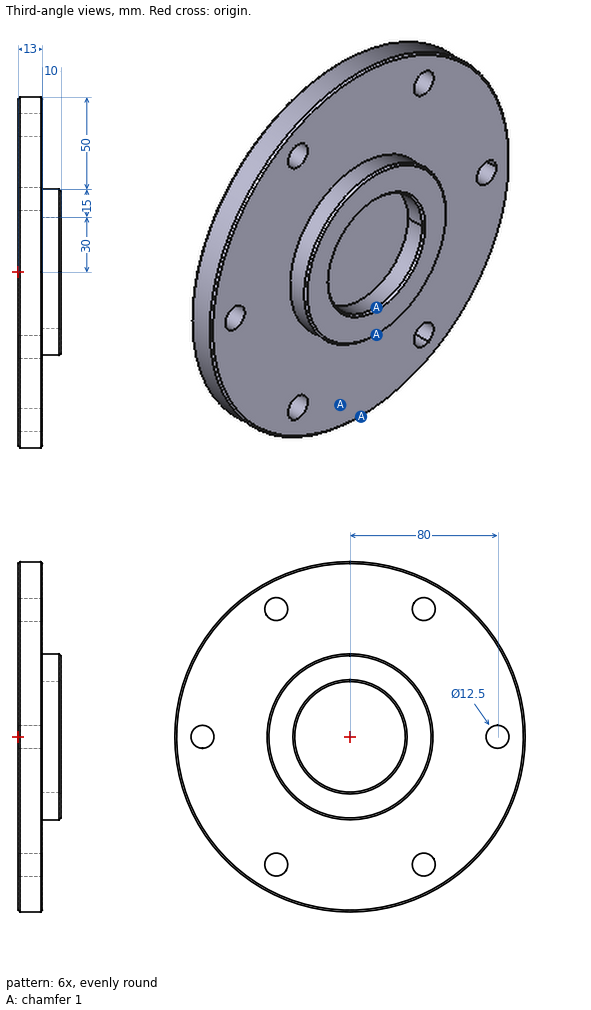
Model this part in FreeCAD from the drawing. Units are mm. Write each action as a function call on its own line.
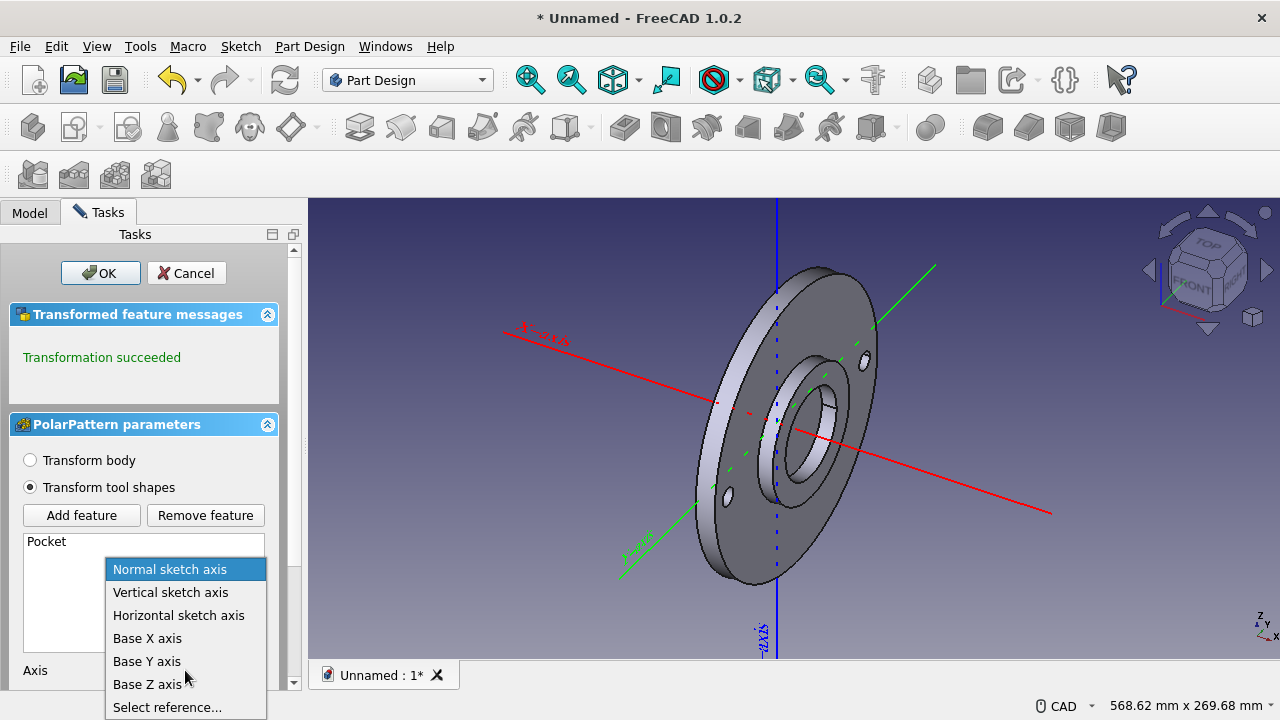
click(184, 638)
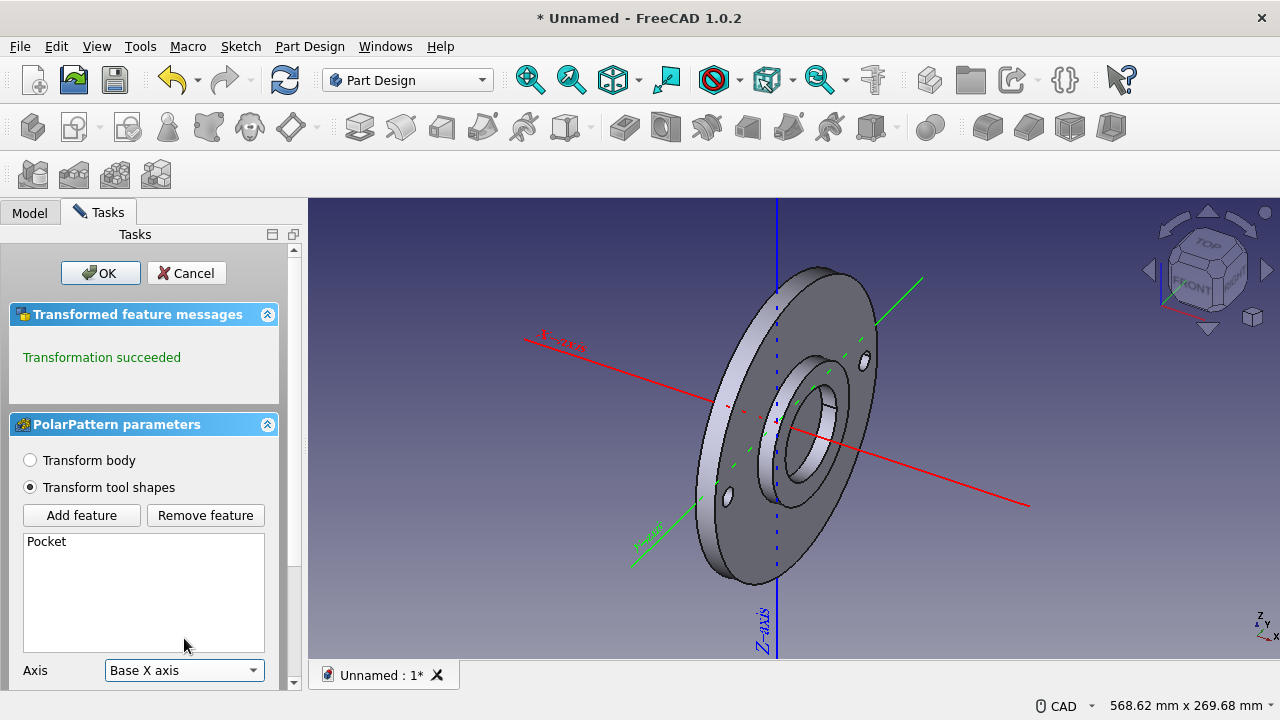
scroll(294, 467, down, 3)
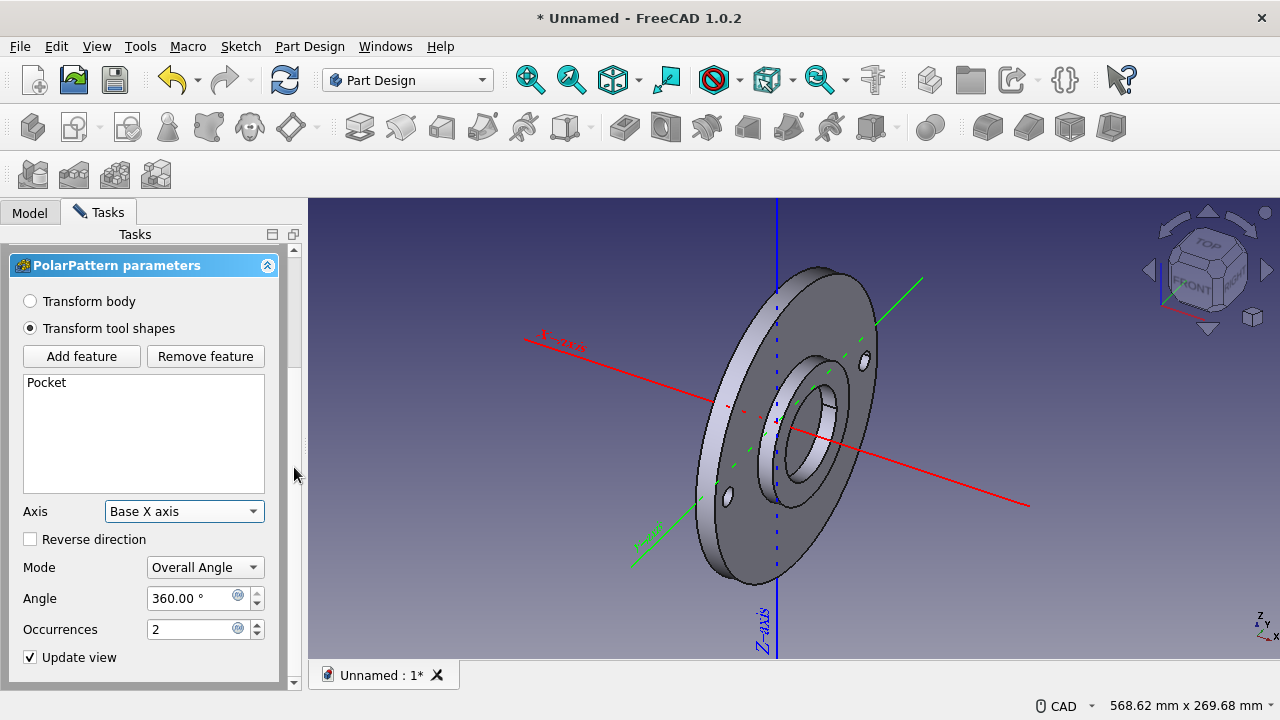
triple_click(199, 630)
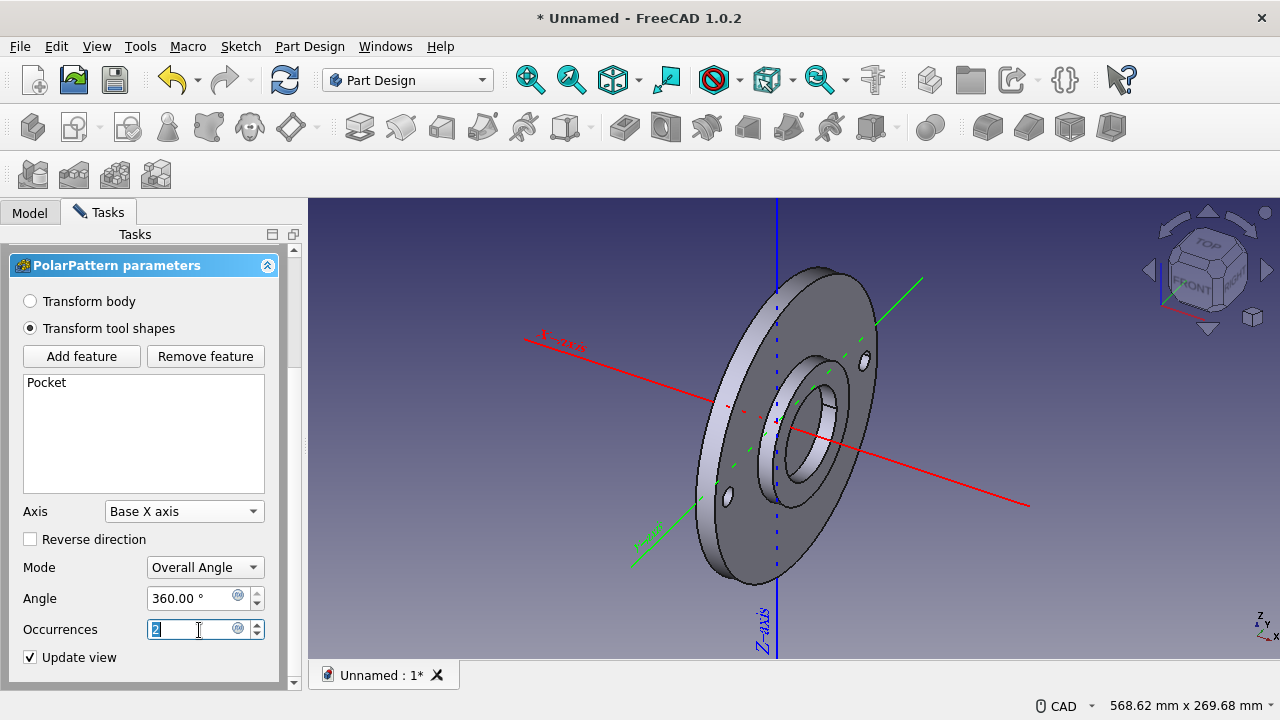
text(6)
key(Tab)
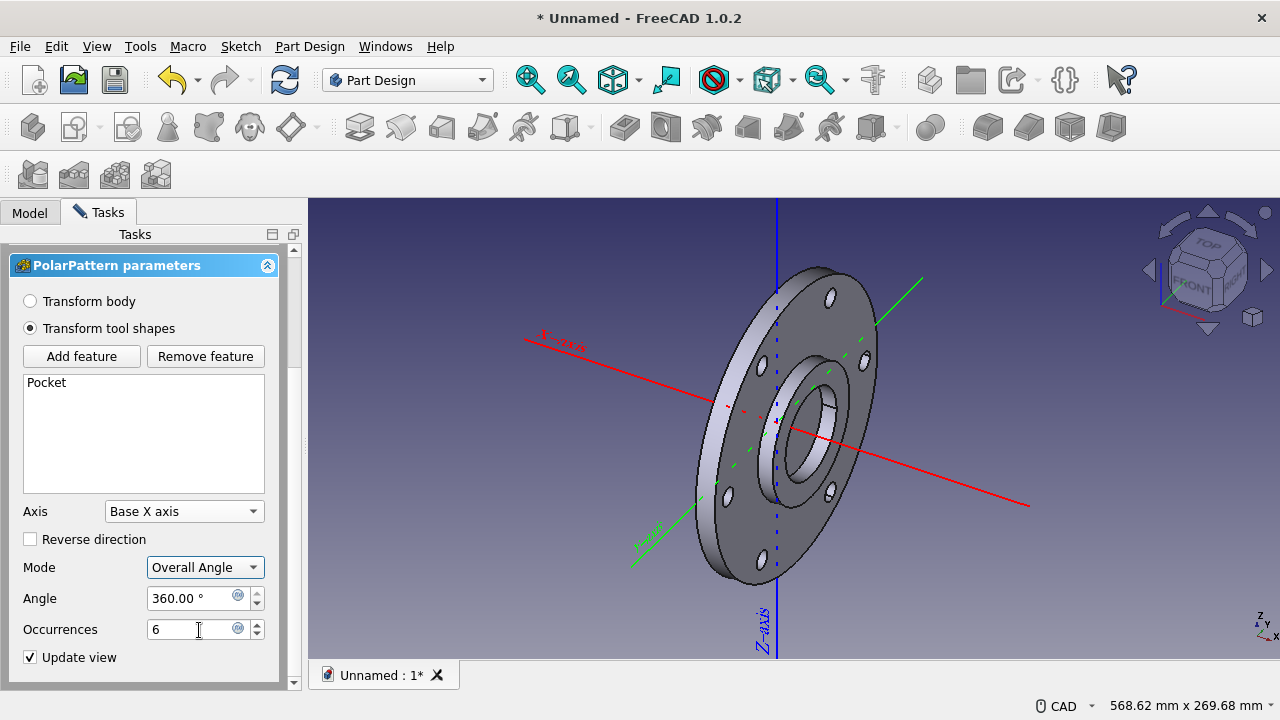
scroll(294, 467, up, 4)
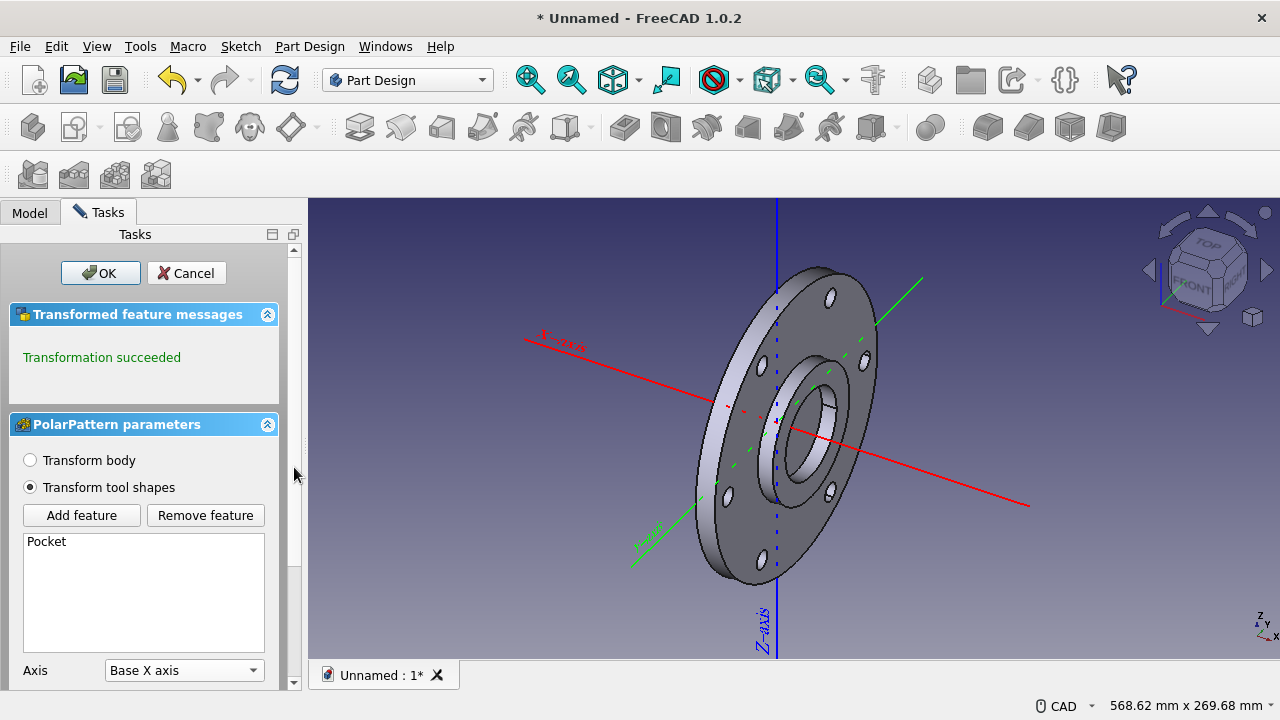
click(101, 273)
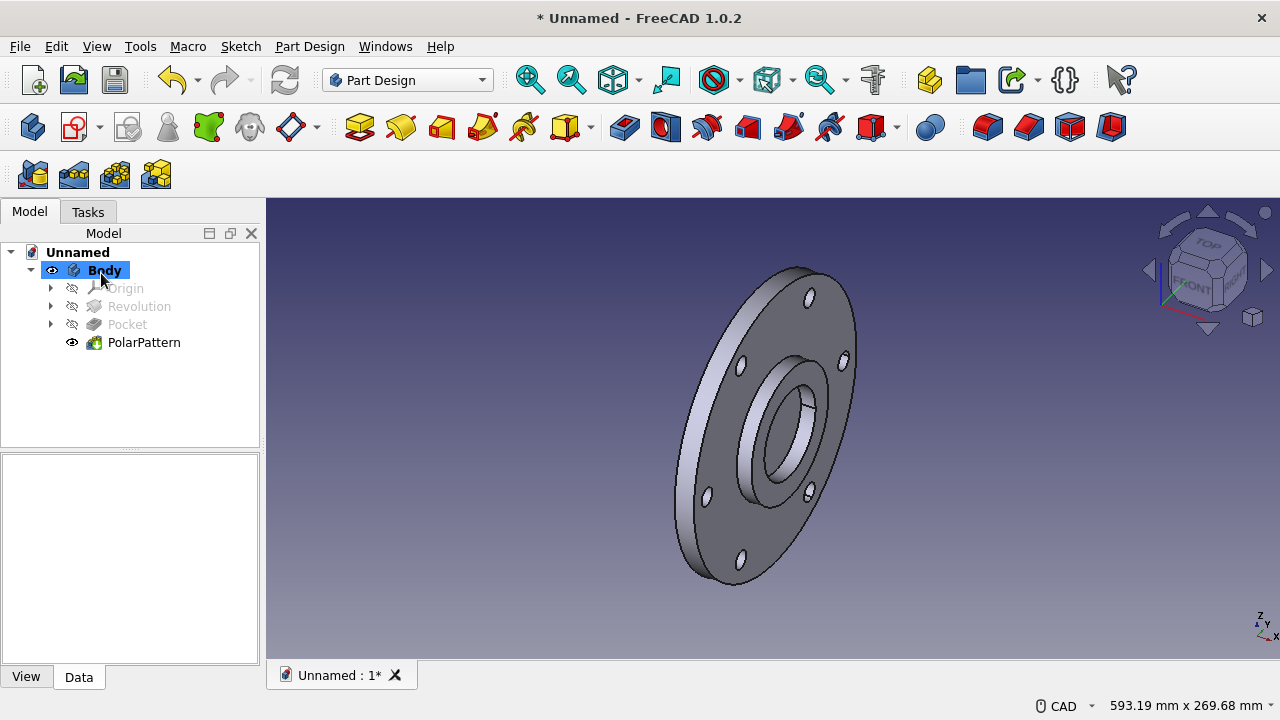
click(782, 481)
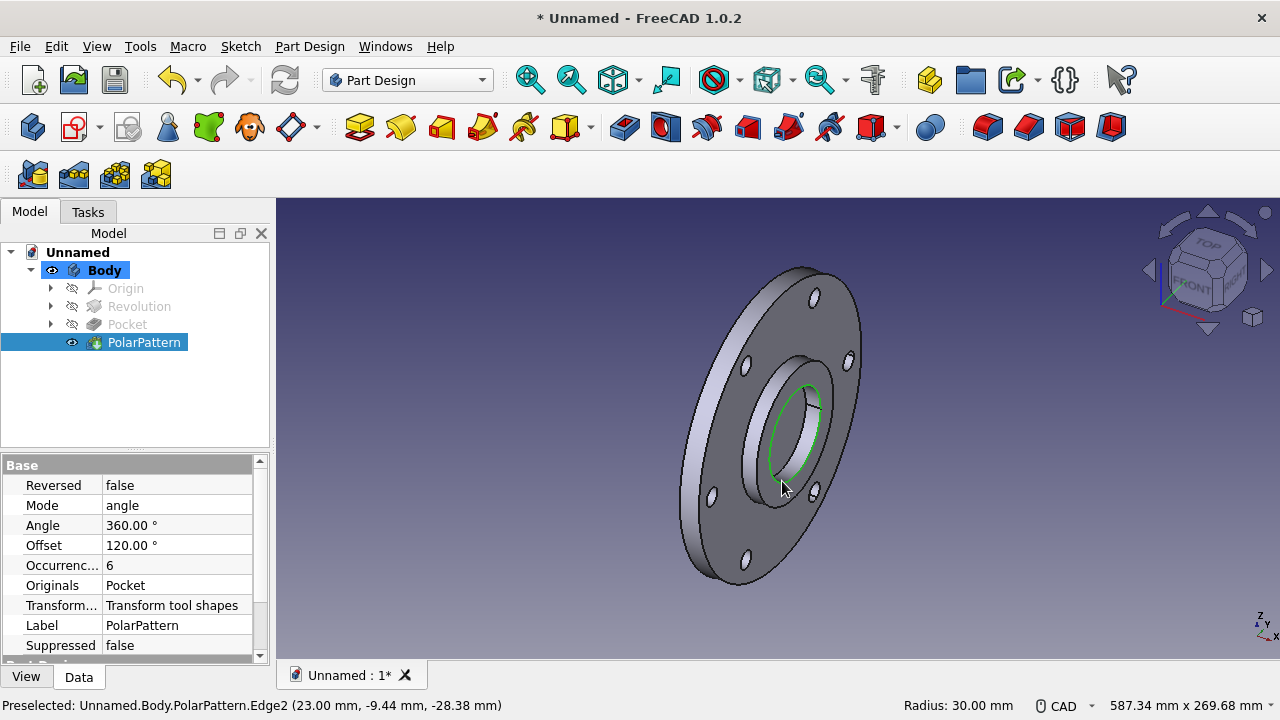
click(757, 471, ctrl)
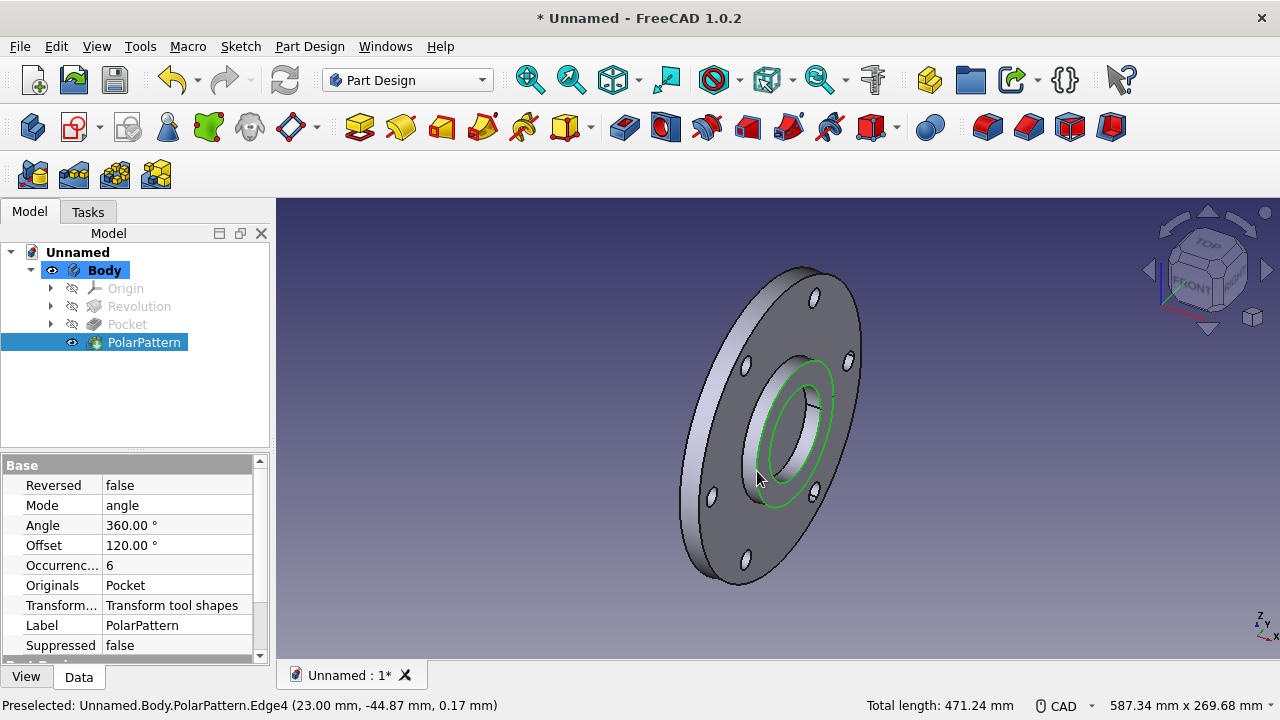
click(699, 509, ctrl)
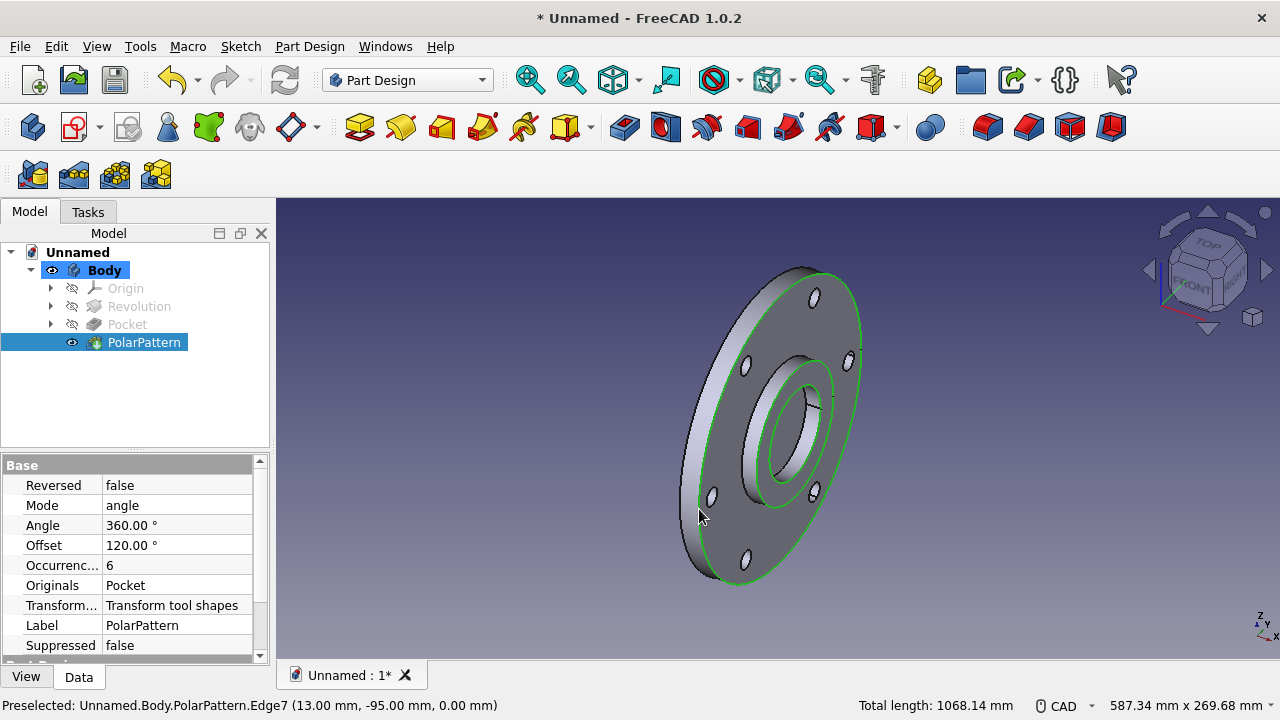
key(0)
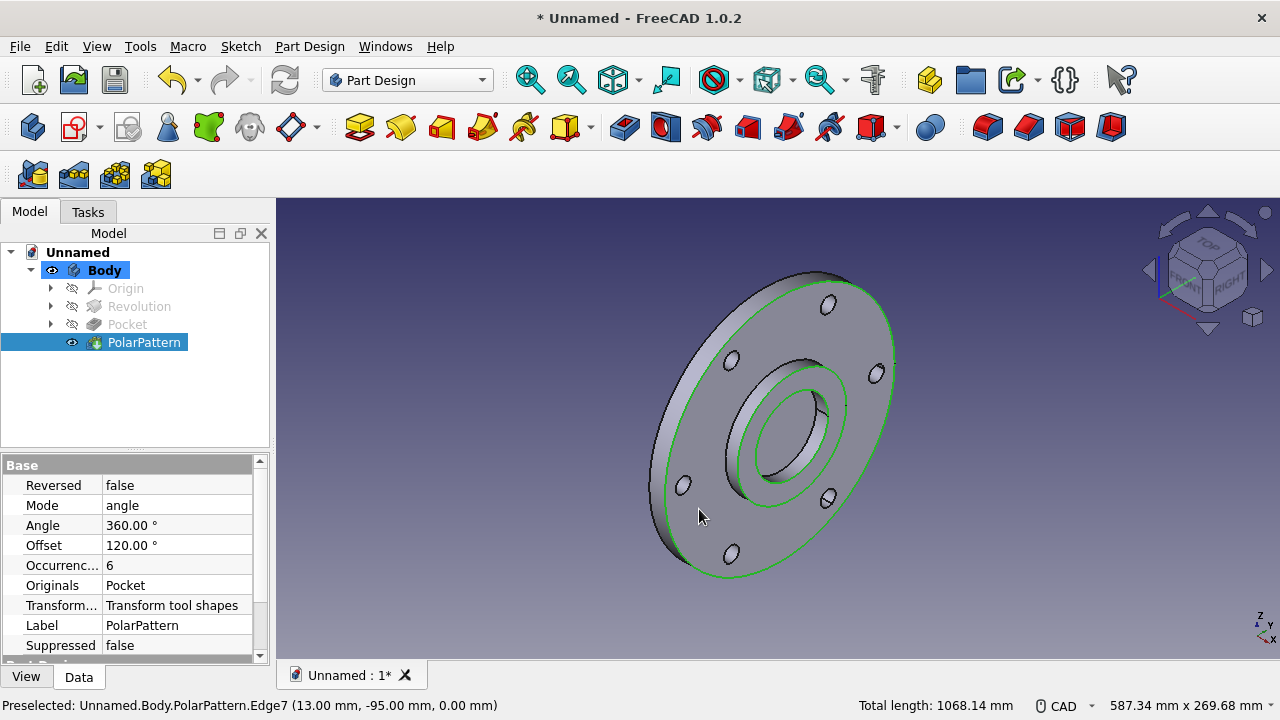
key(2)